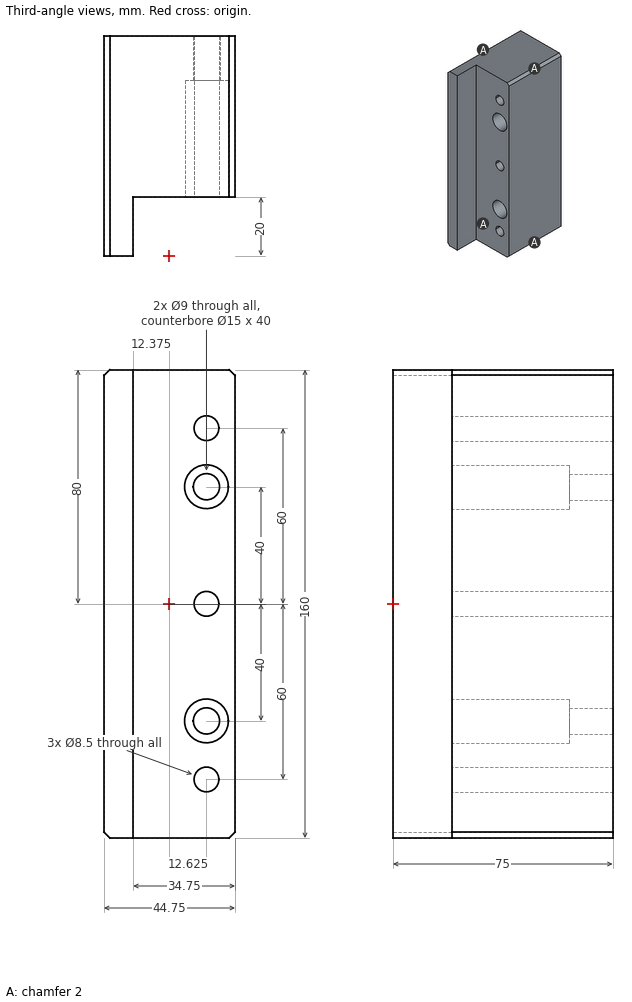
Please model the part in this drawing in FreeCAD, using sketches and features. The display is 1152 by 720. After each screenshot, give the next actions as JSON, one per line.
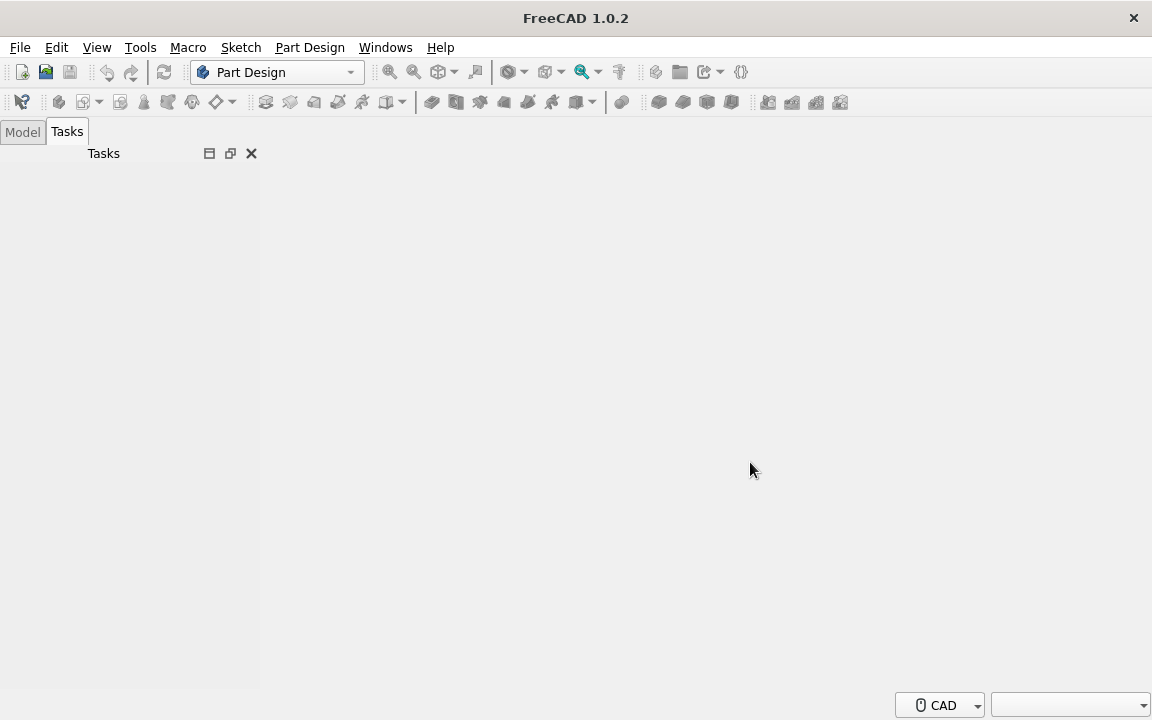
{"action": "left_click", "coordinate": [22, 72]}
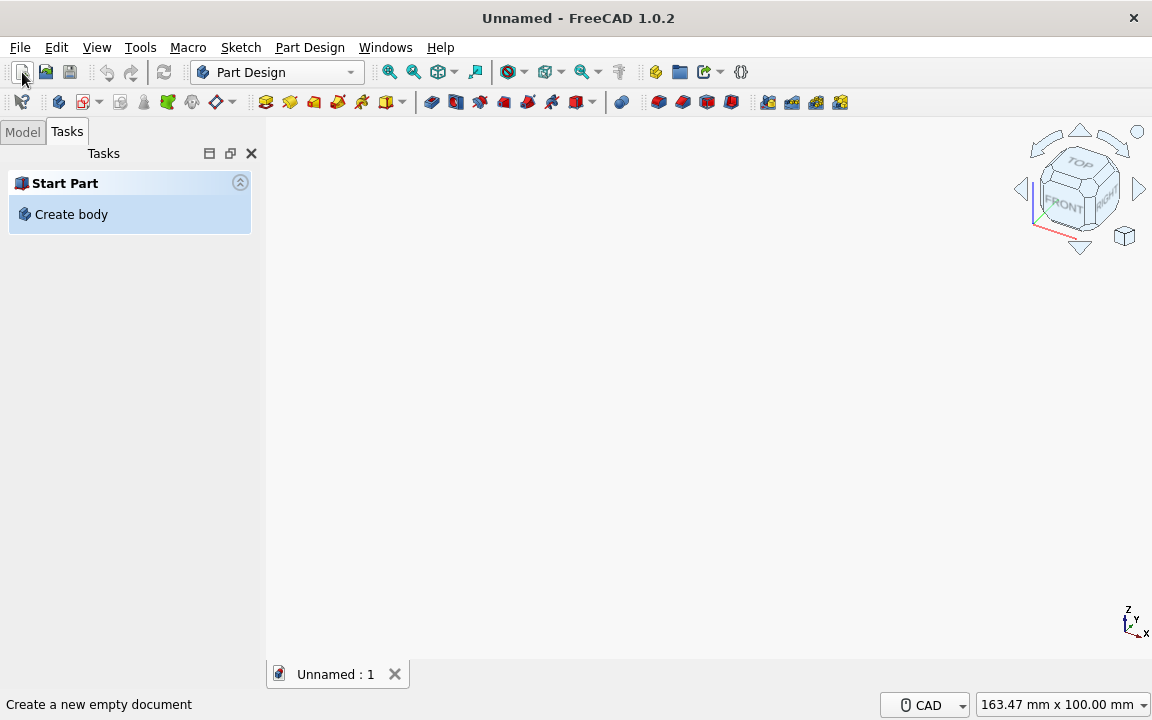
{"action": "left_click", "coordinate": [84, 102]}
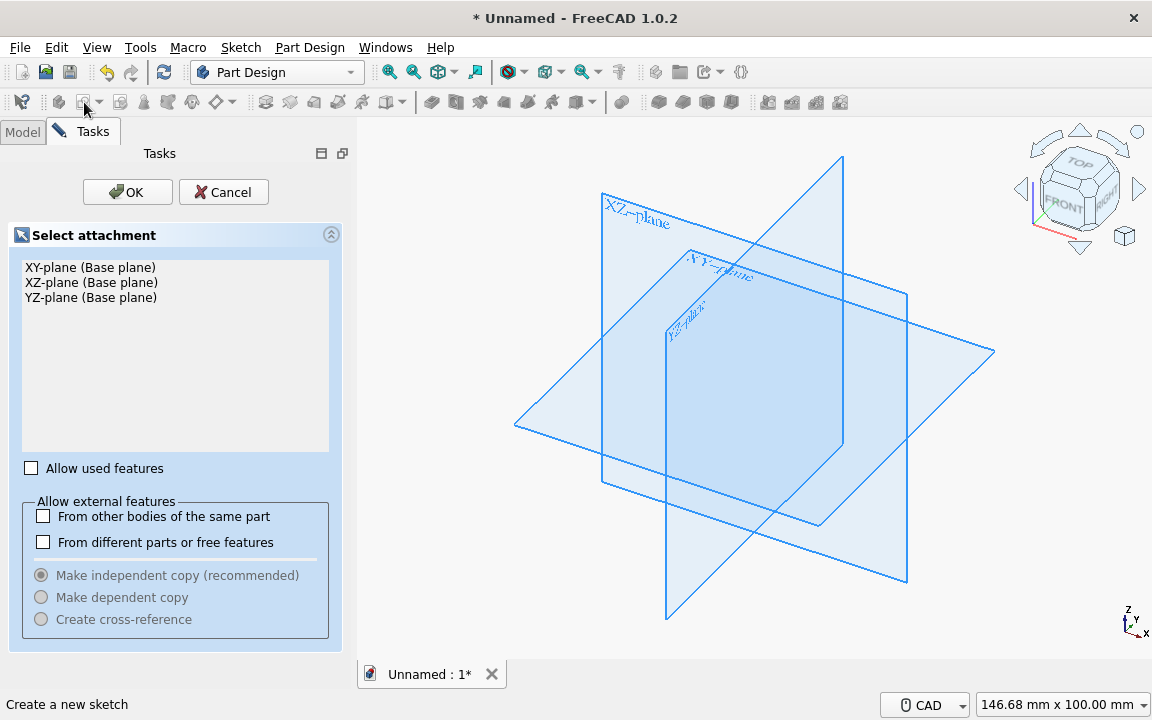
{"action": "left_click", "coordinate": [82, 282]}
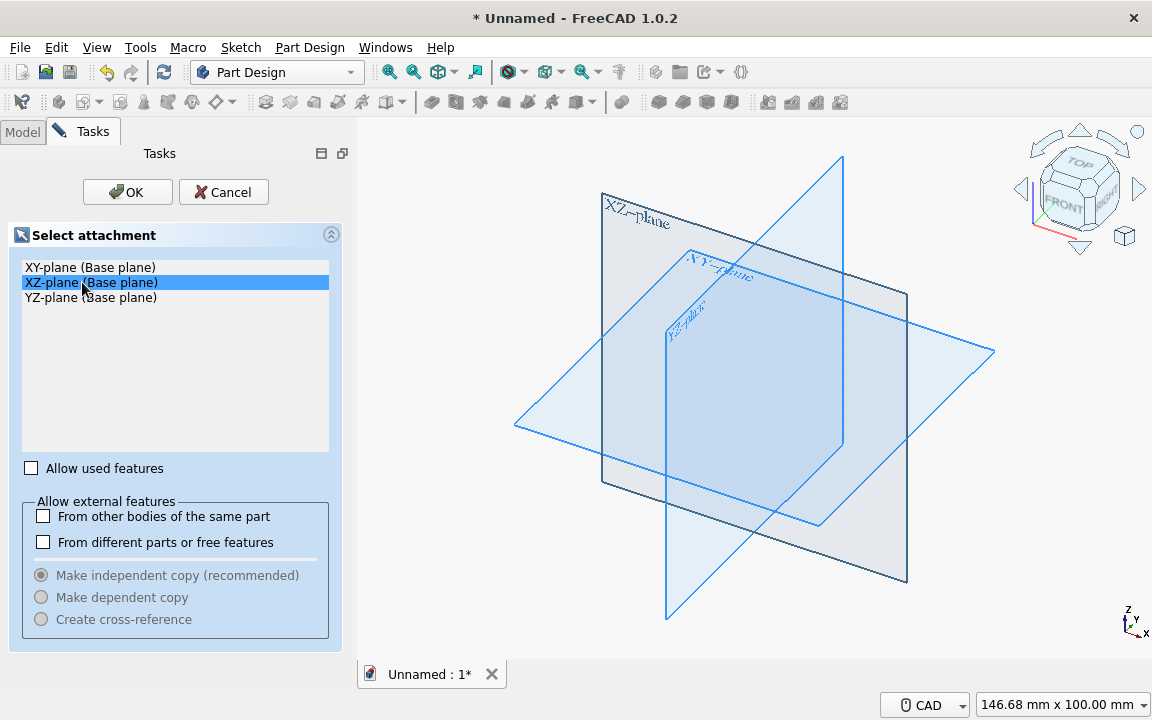
{"action": "left_click", "coordinate": [128, 192]}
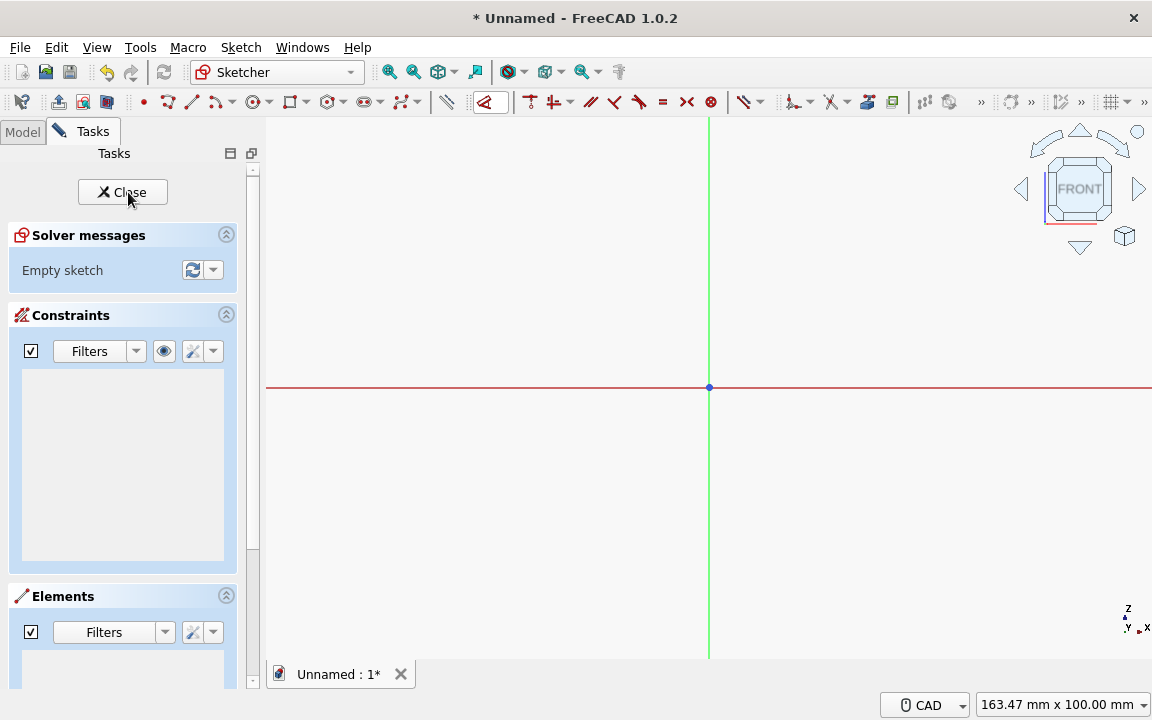
{"action": "scroll", "coordinate": [601, 388], "scroll_direction": "down", "scroll_amount": 5}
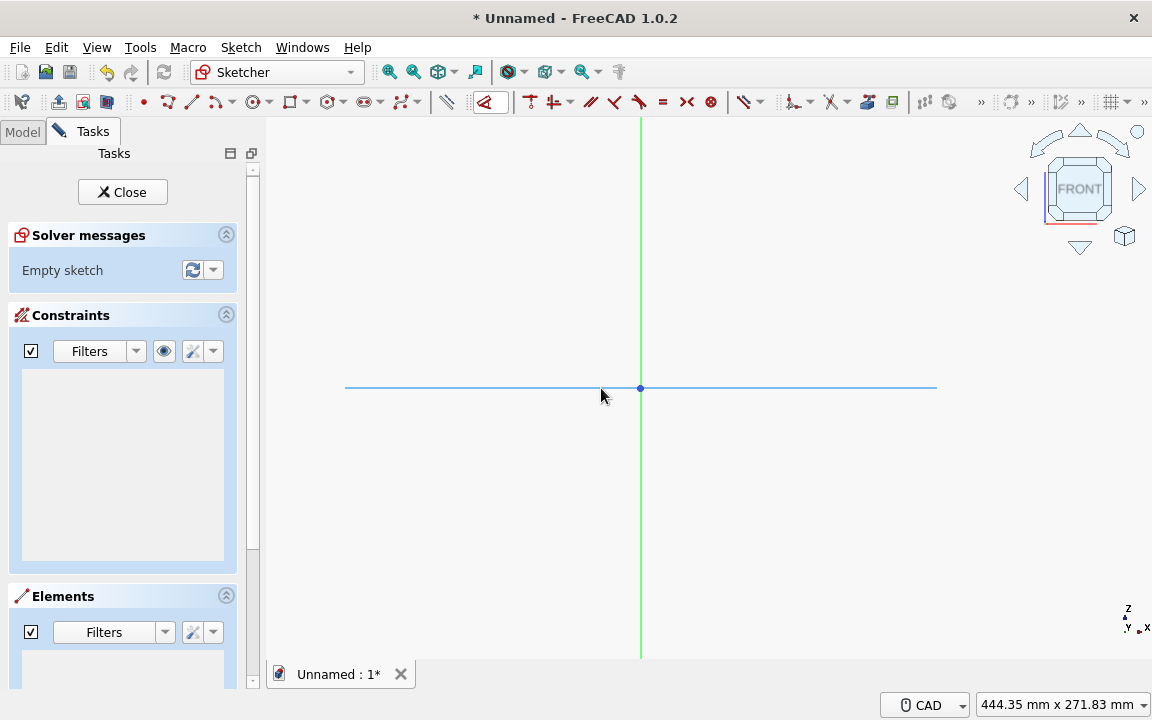
{"action": "left_click", "coordinate": [308, 102]}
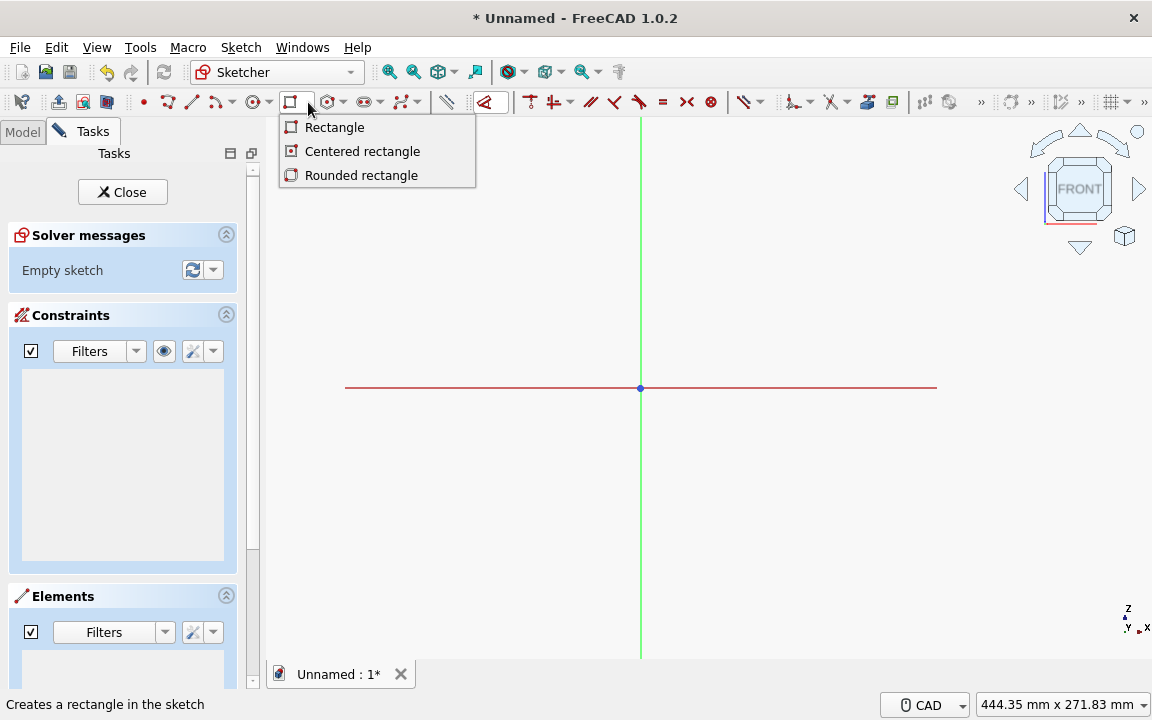
{"action": "left_click", "coordinate": [378, 151]}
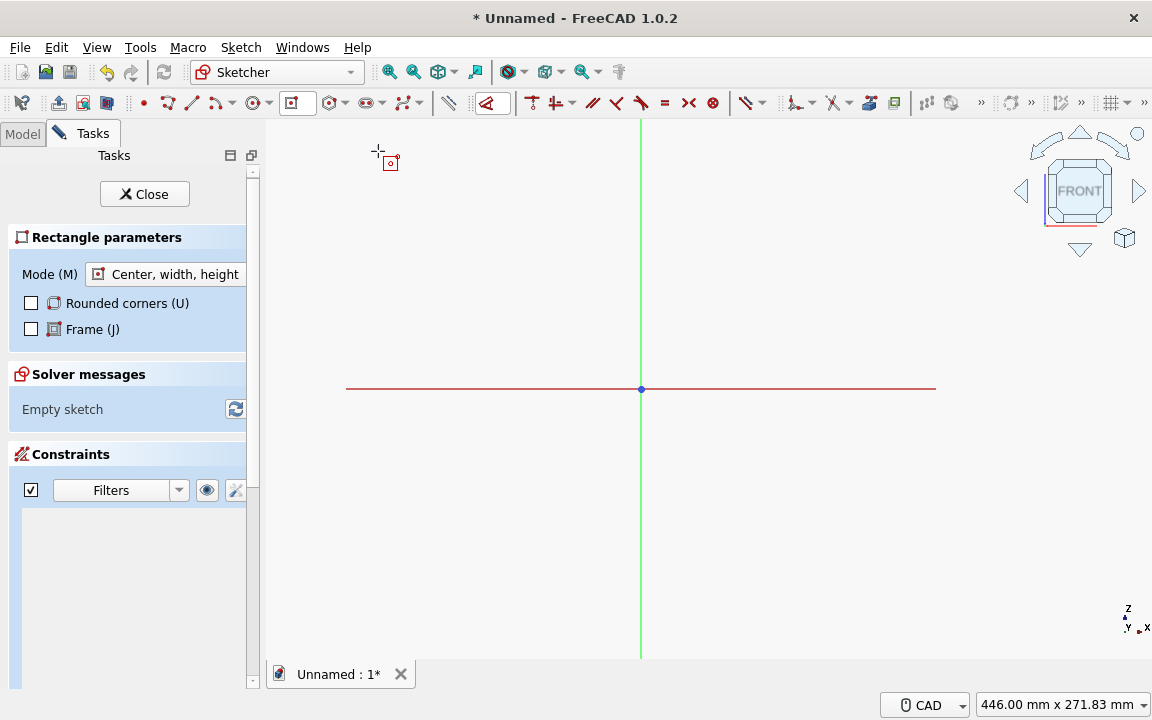
{"action": "left_click", "coordinate": [641, 389]}
{"action": "left_click", "coordinate": [686, 230]}
{"action": "key", "text": "Escape"}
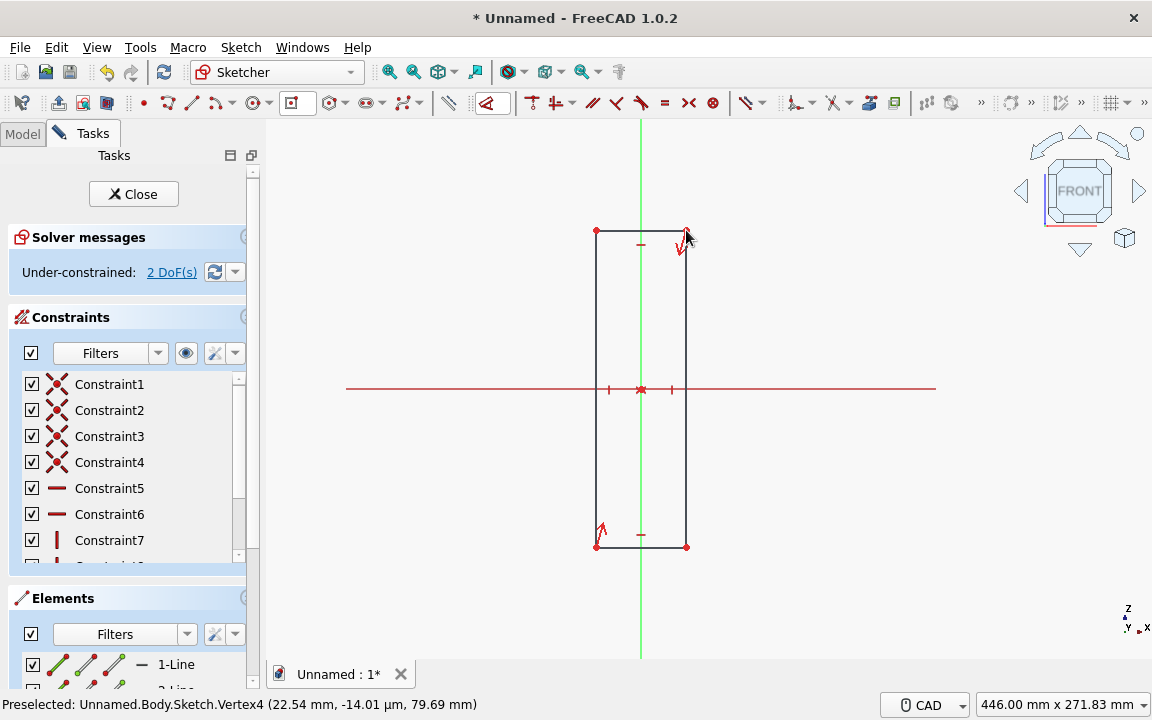
{"action": "key", "text": "d"}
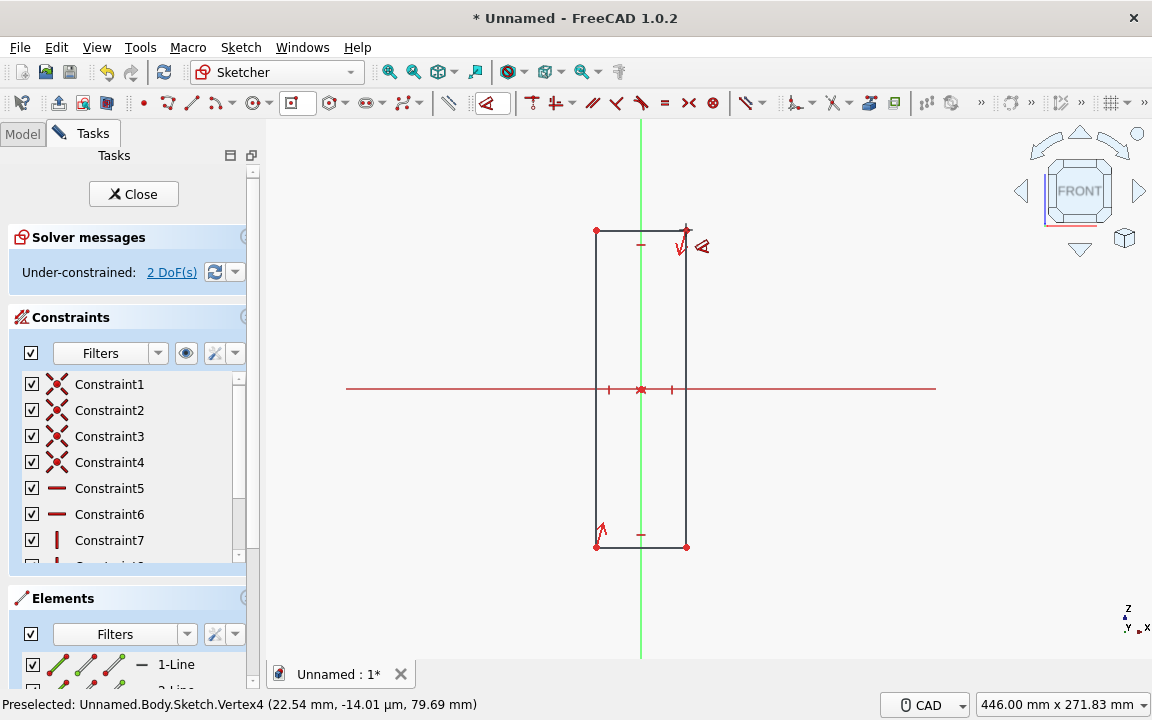
{"action": "left_click", "coordinate": [686, 453]}
{"action": "left_click", "coordinate": [720, 316]}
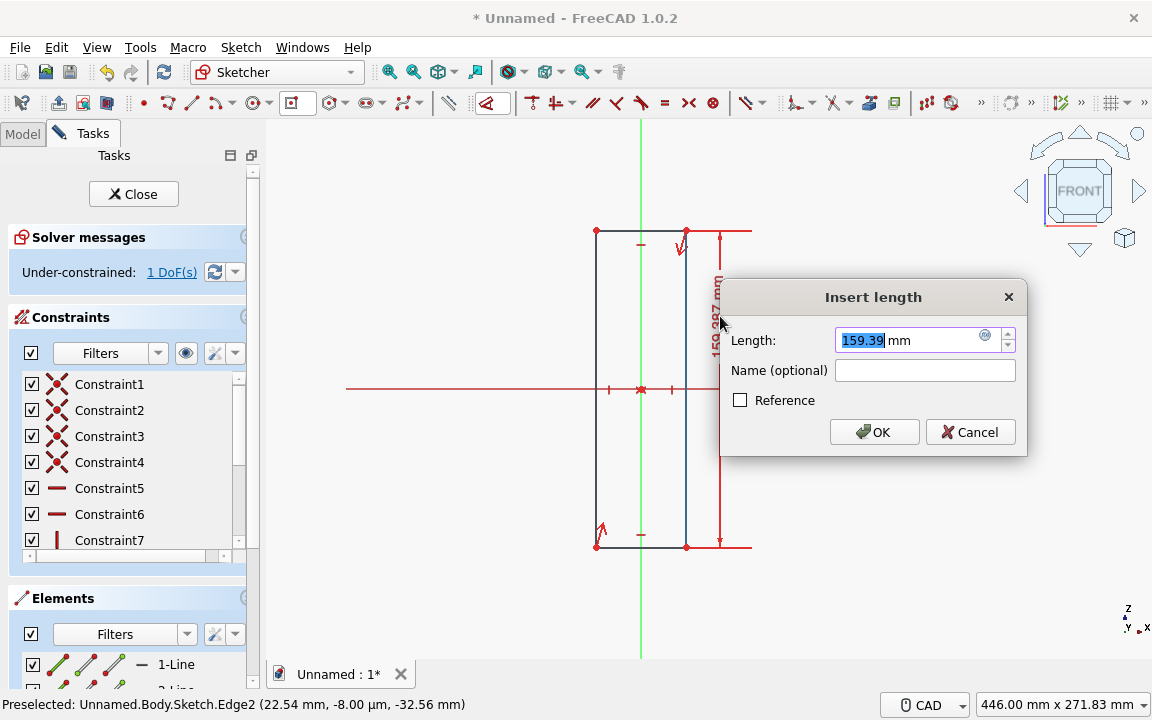
{"action": "type", "text": "160"}
{"action": "key", "text": "Return"}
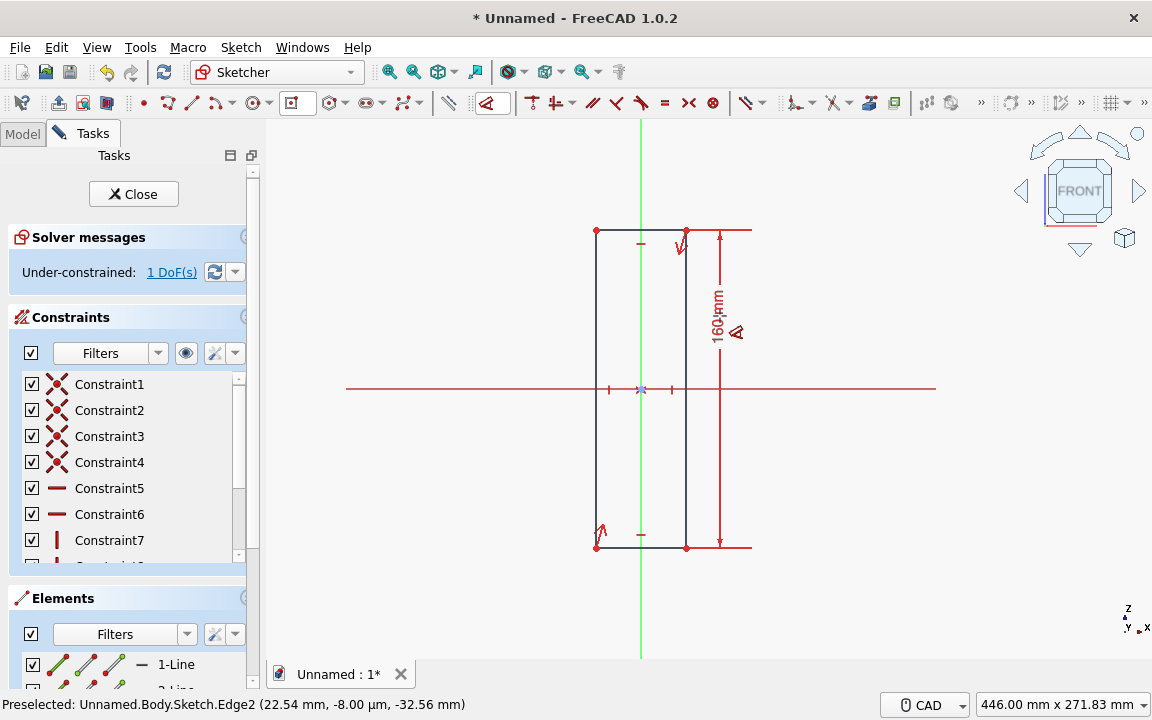
{"action": "left_click", "coordinate": [623, 548]}
{"action": "left_click", "coordinate": [621, 582]}